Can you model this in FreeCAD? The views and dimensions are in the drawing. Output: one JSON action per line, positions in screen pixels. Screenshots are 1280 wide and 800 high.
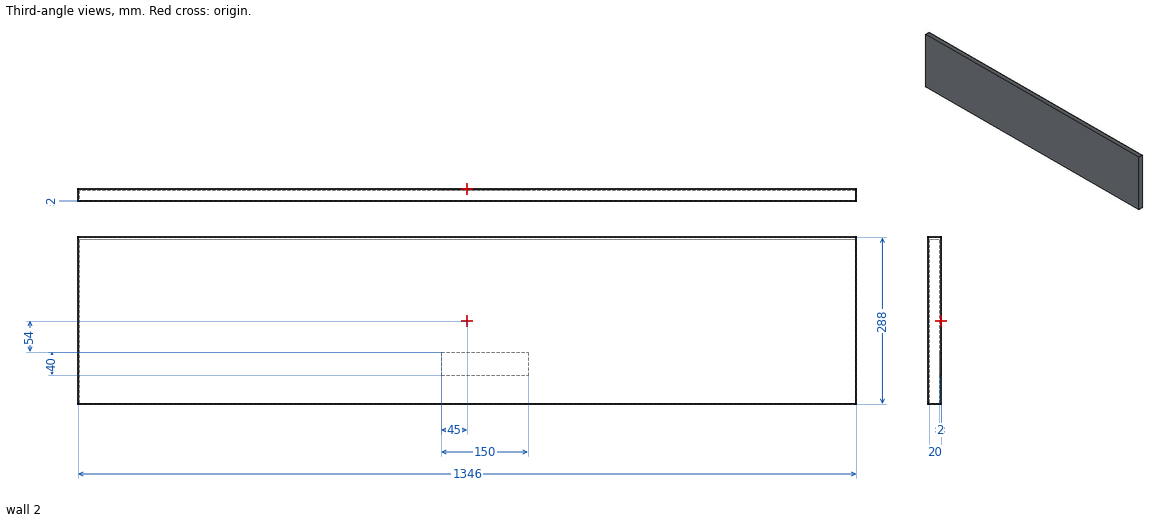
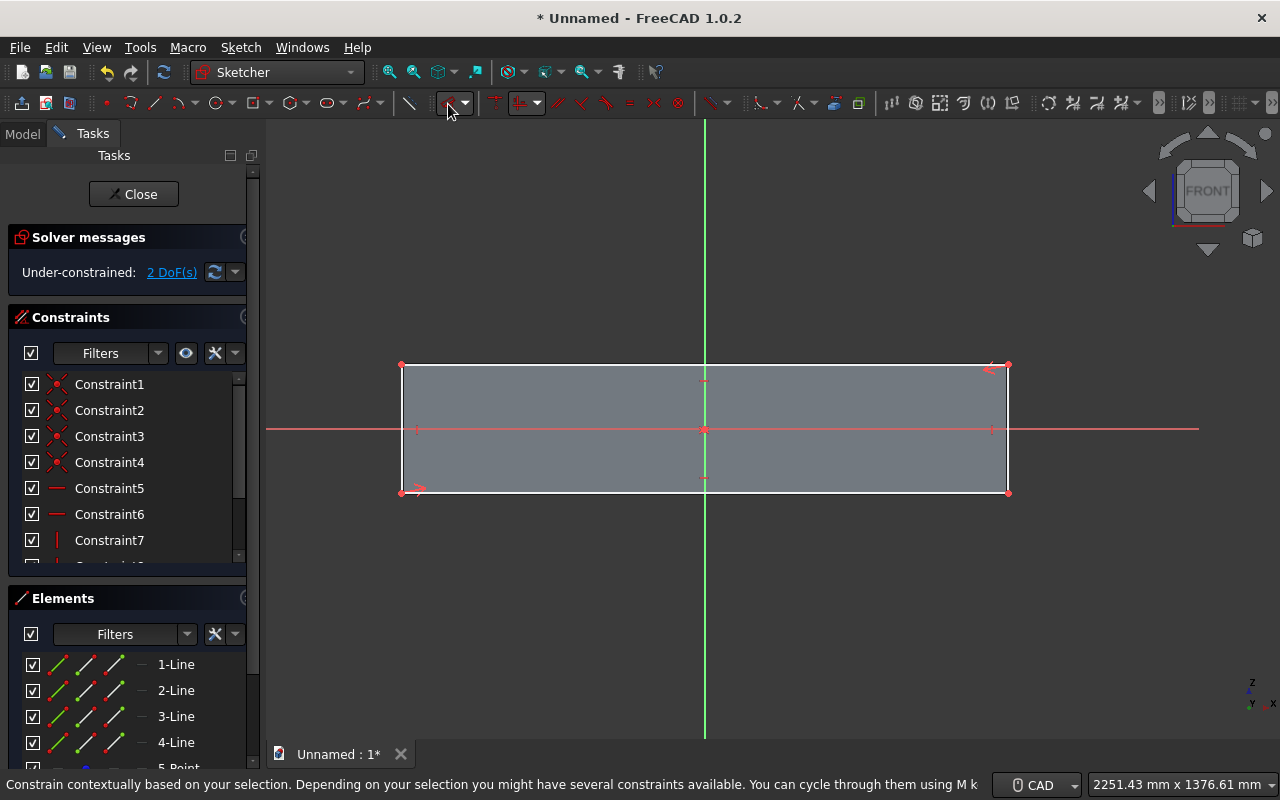
{"action": "left_click", "coordinate": [1008, 455]}
{"action": "left_click", "coordinate": [1042, 400]}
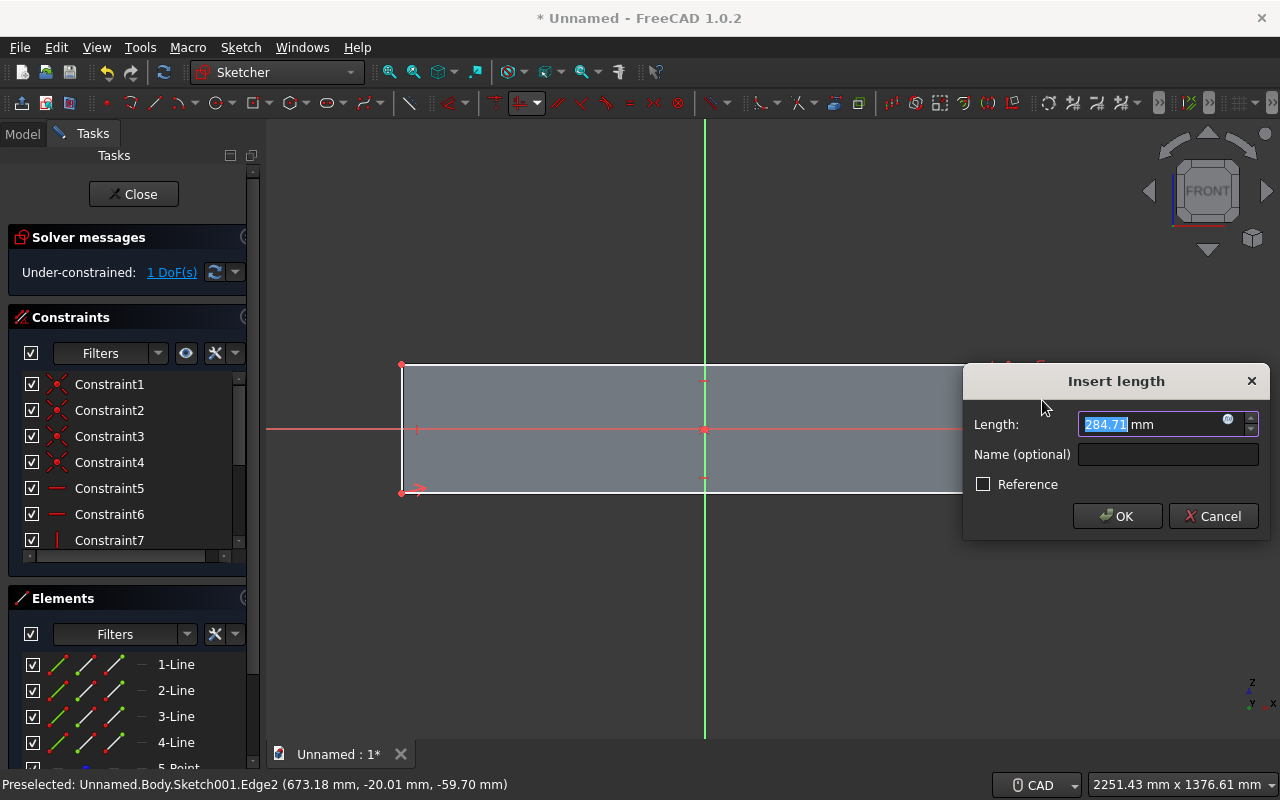
{"action": "type", "text": "288"}
{"action": "key", "text": "Return"}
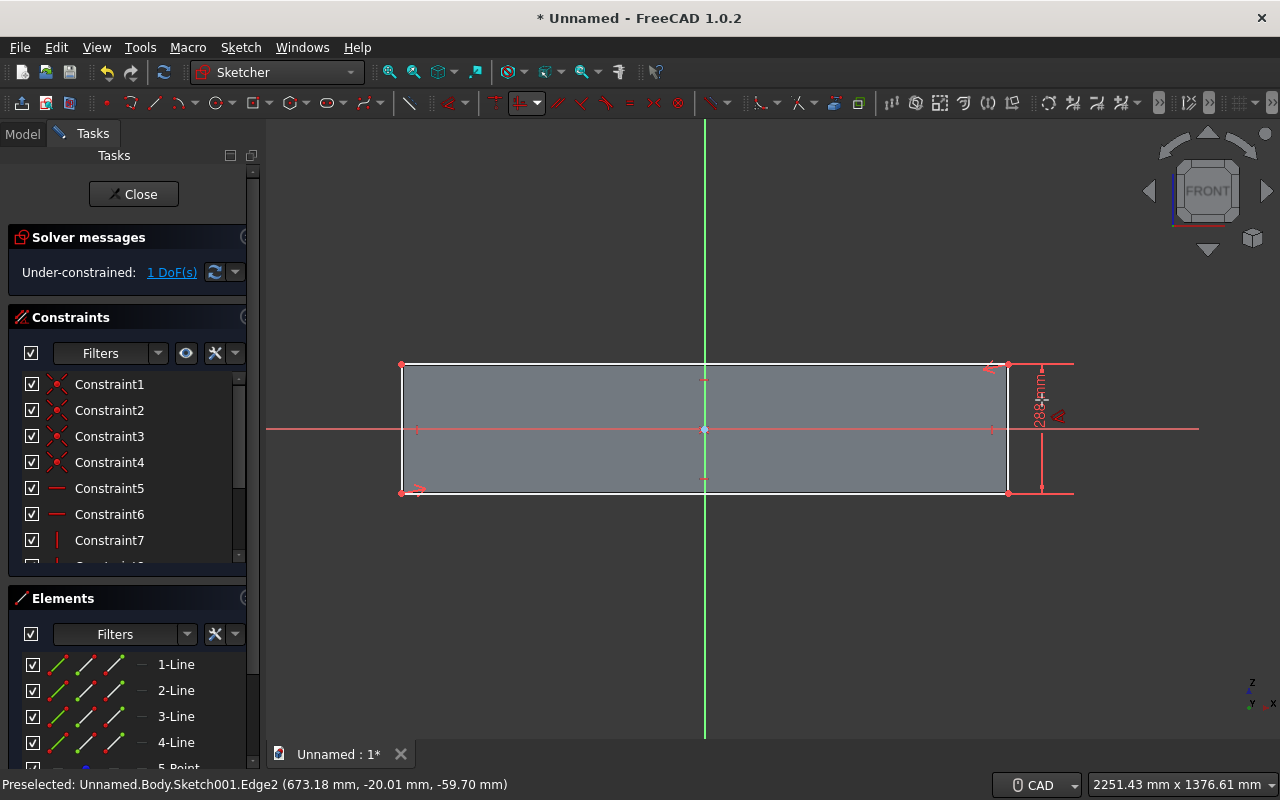
{"action": "left_click", "coordinate": [584, 494]}
{"action": "left_click", "coordinate": [565, 528]}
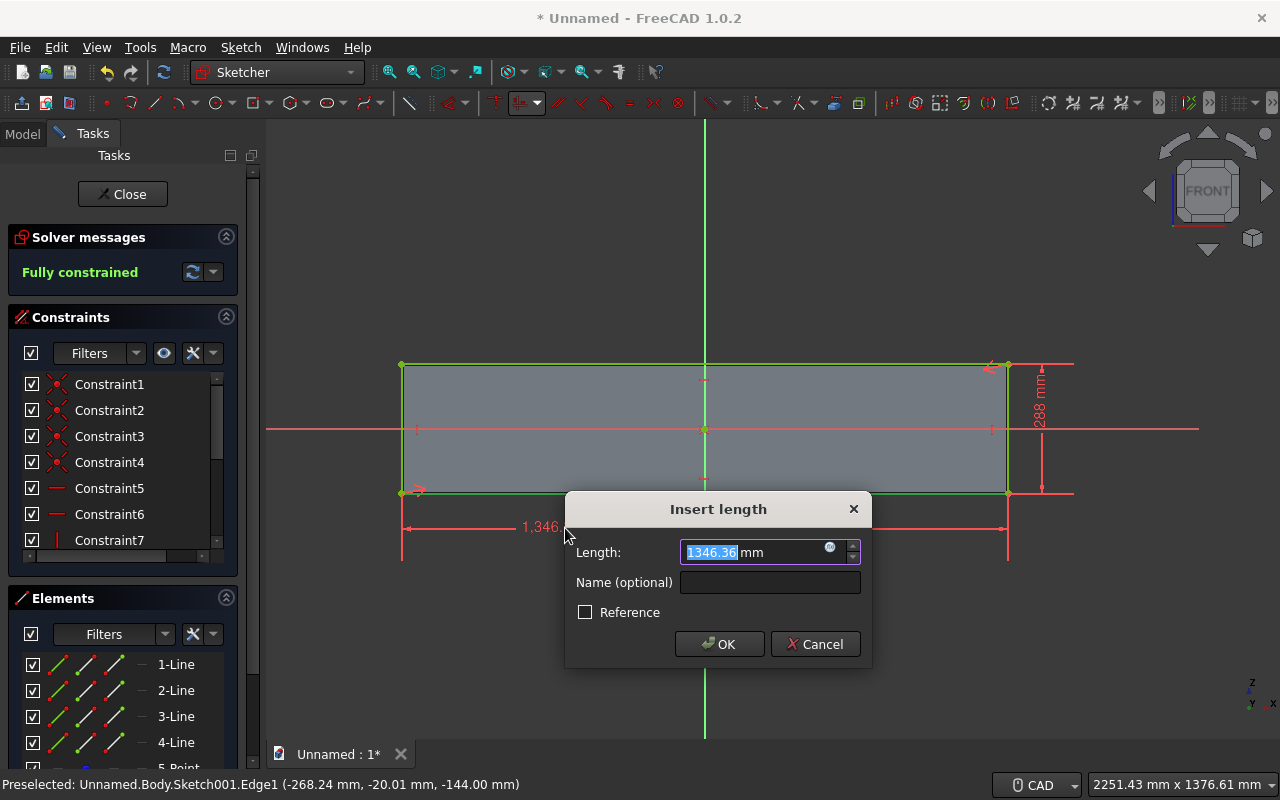
{"action": "type", "text": "1346"}
{"action": "key", "text": "Return"}
{"action": "key", "text": "Escape"}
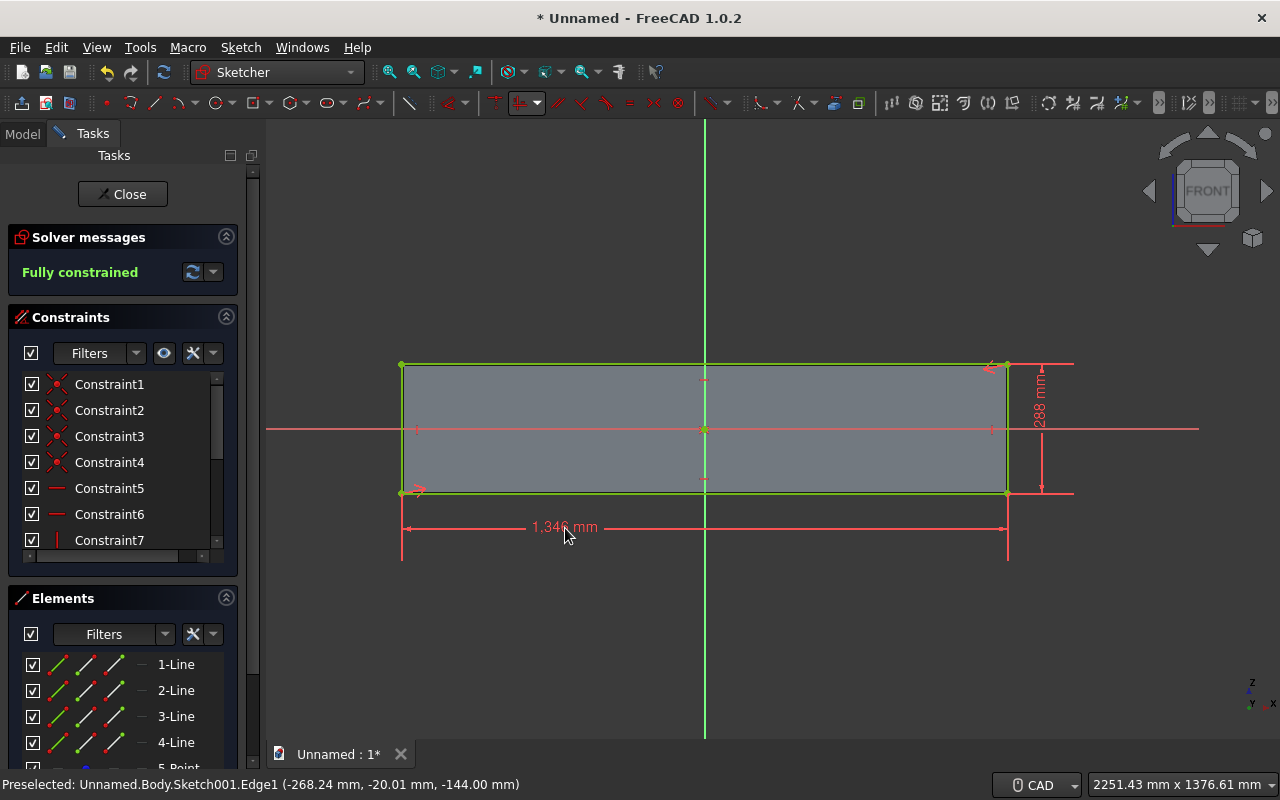
{"action": "left_click", "coordinate": [123, 194]}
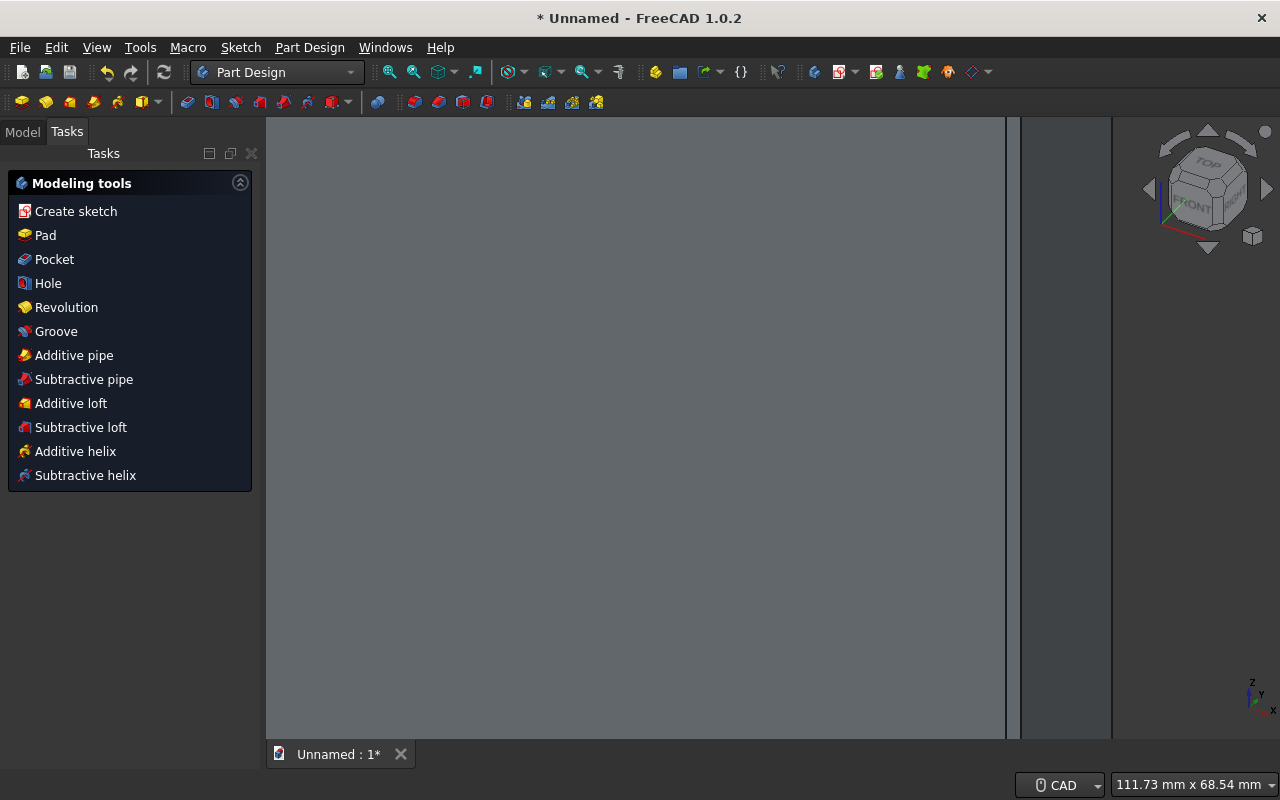
{"action": "left_click", "coordinate": [22, 102]}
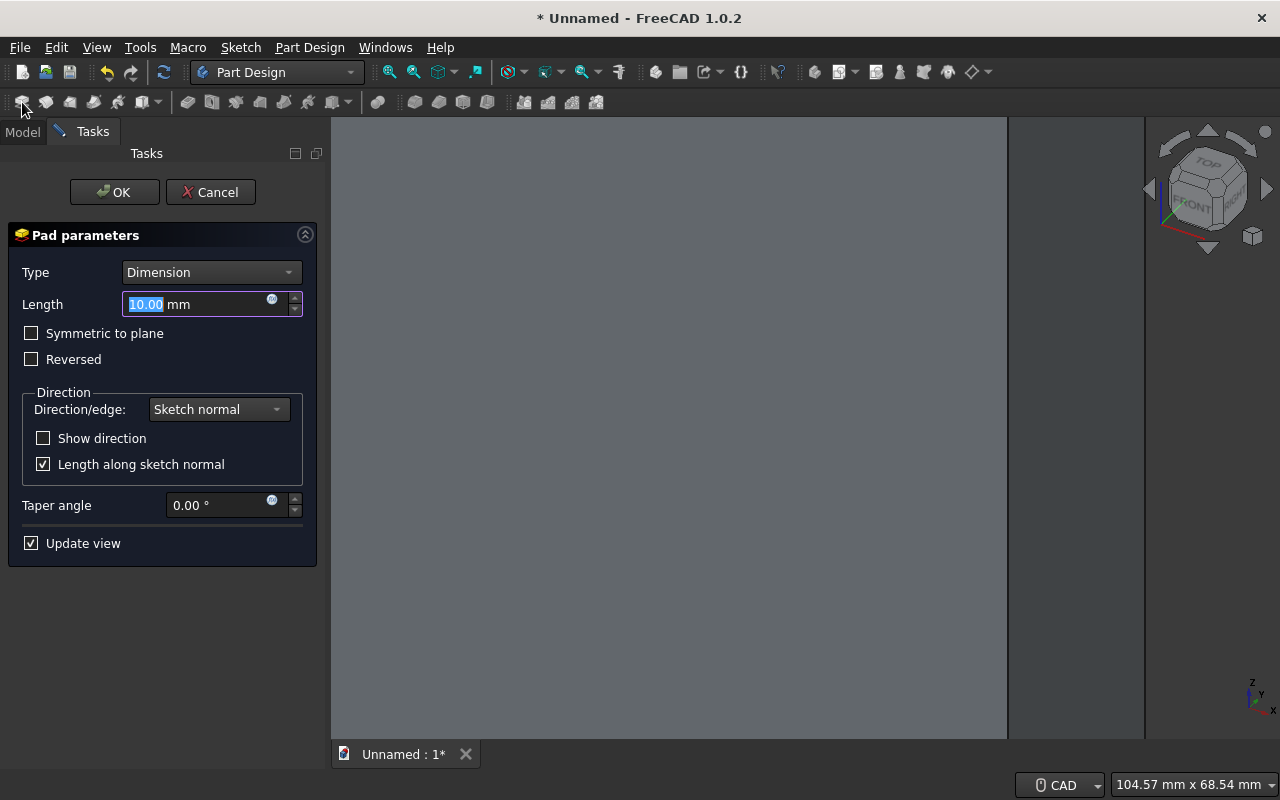
{"action": "type", "text": "2"}
{"action": "key", "text": "Tab"}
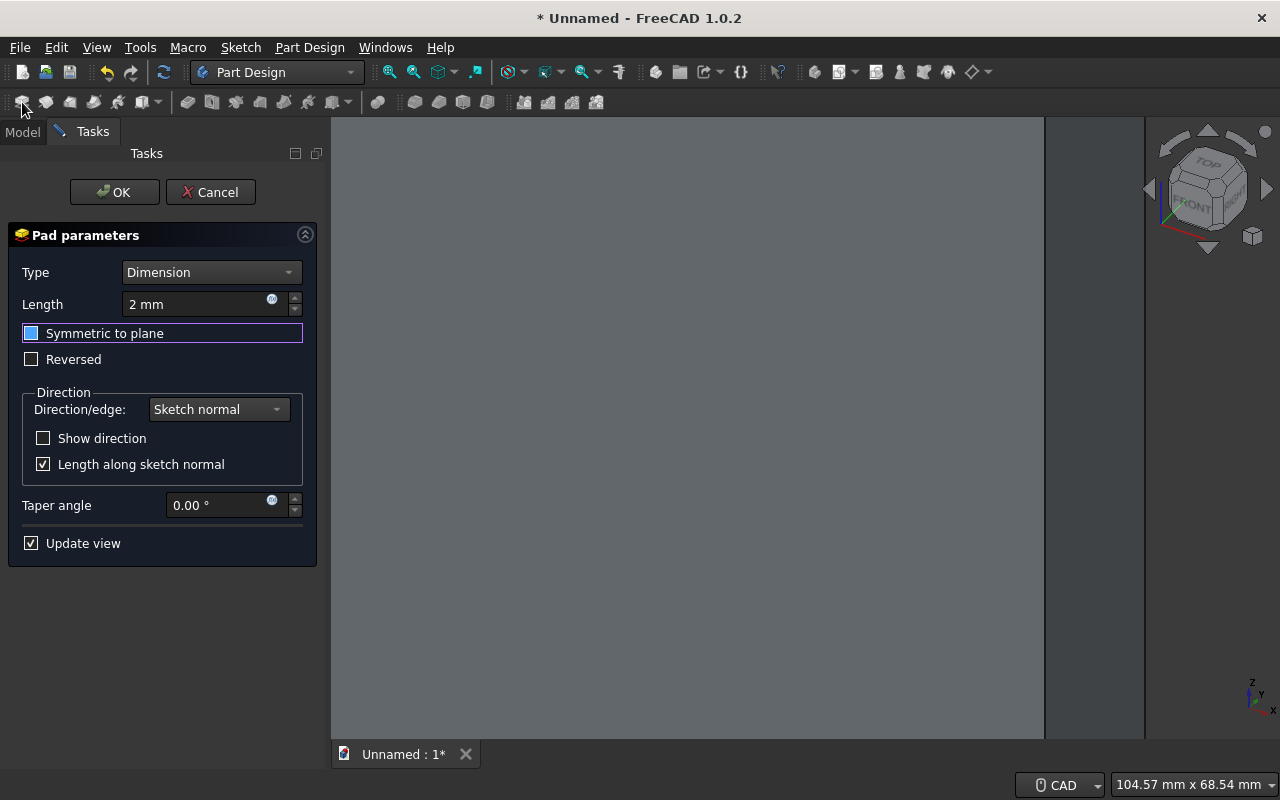
{"action": "left_click", "coordinate": [115, 192]}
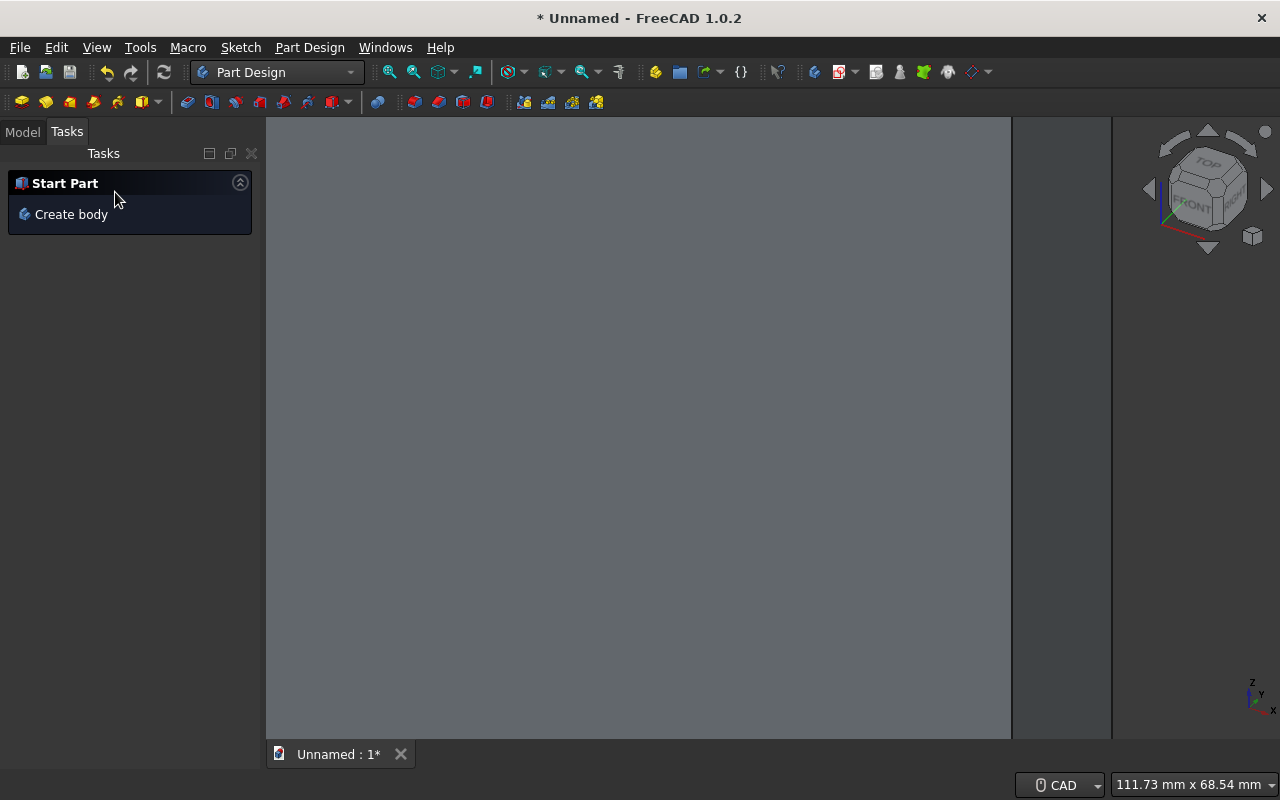
{"action": "key", "text": "v f"}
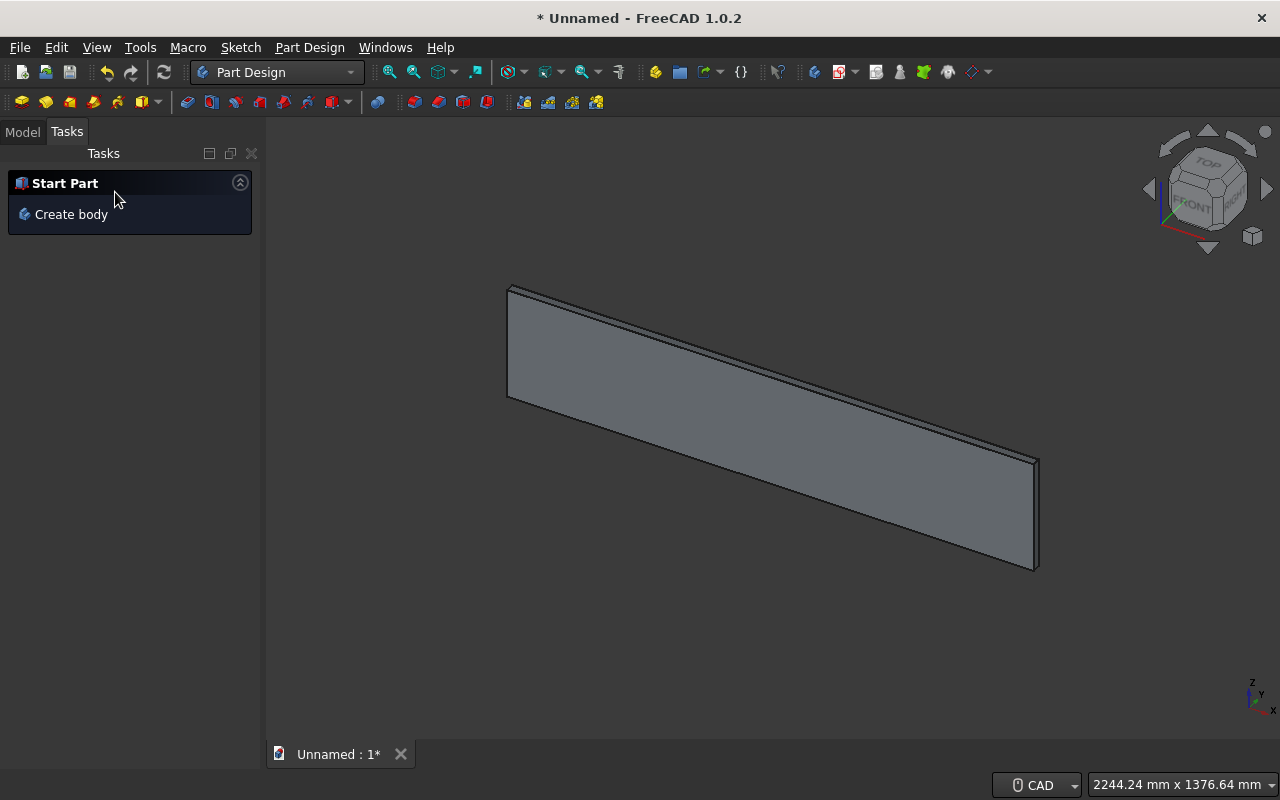
{"action": "left_click", "coordinate": [840, 72]}